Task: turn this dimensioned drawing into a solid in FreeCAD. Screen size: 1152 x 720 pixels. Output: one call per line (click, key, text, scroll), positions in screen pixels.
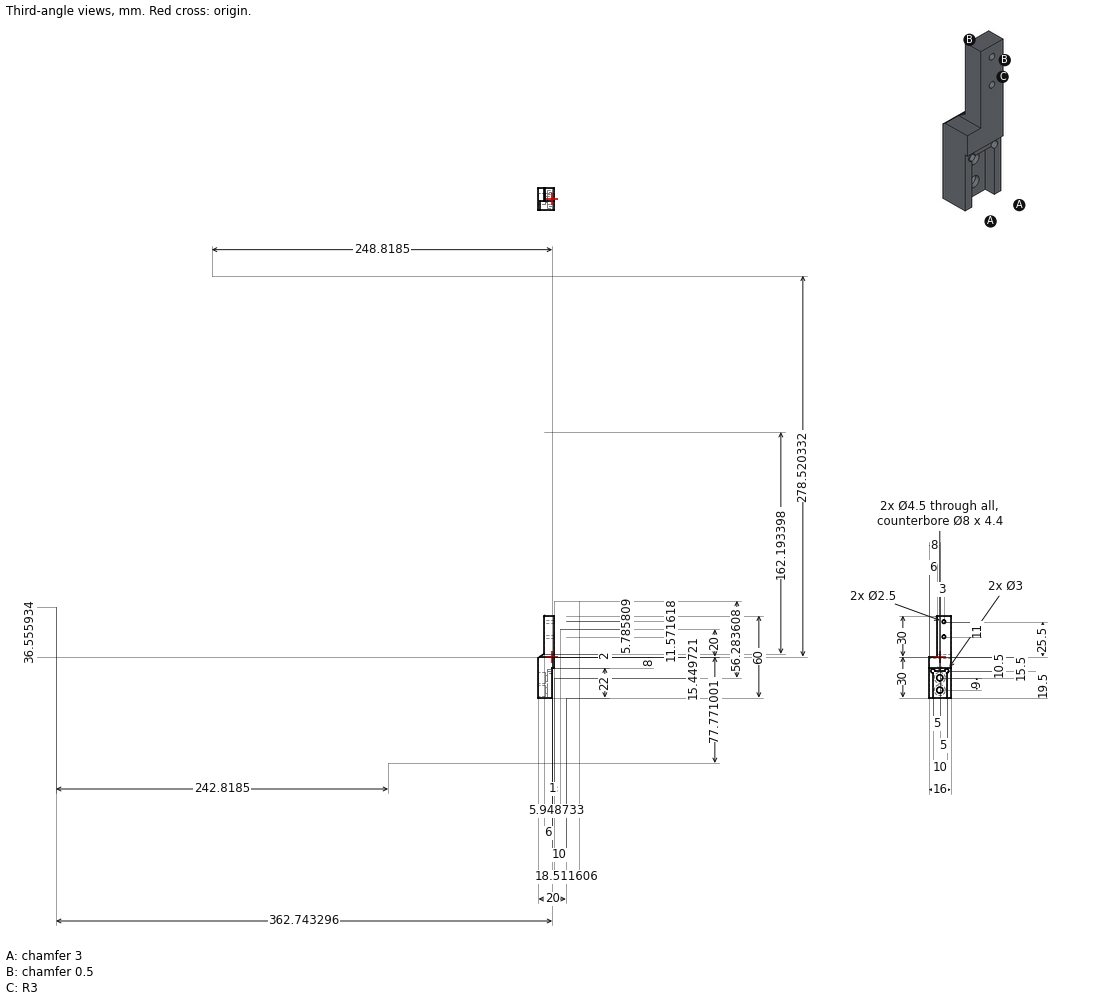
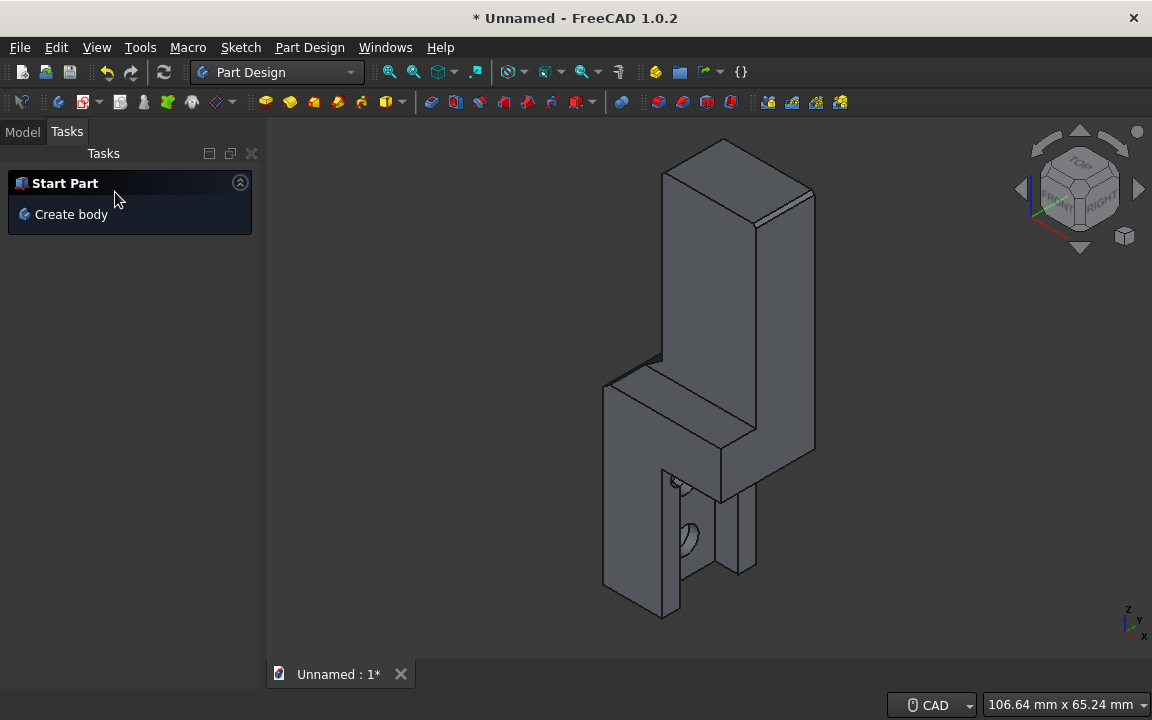
click(716, 303)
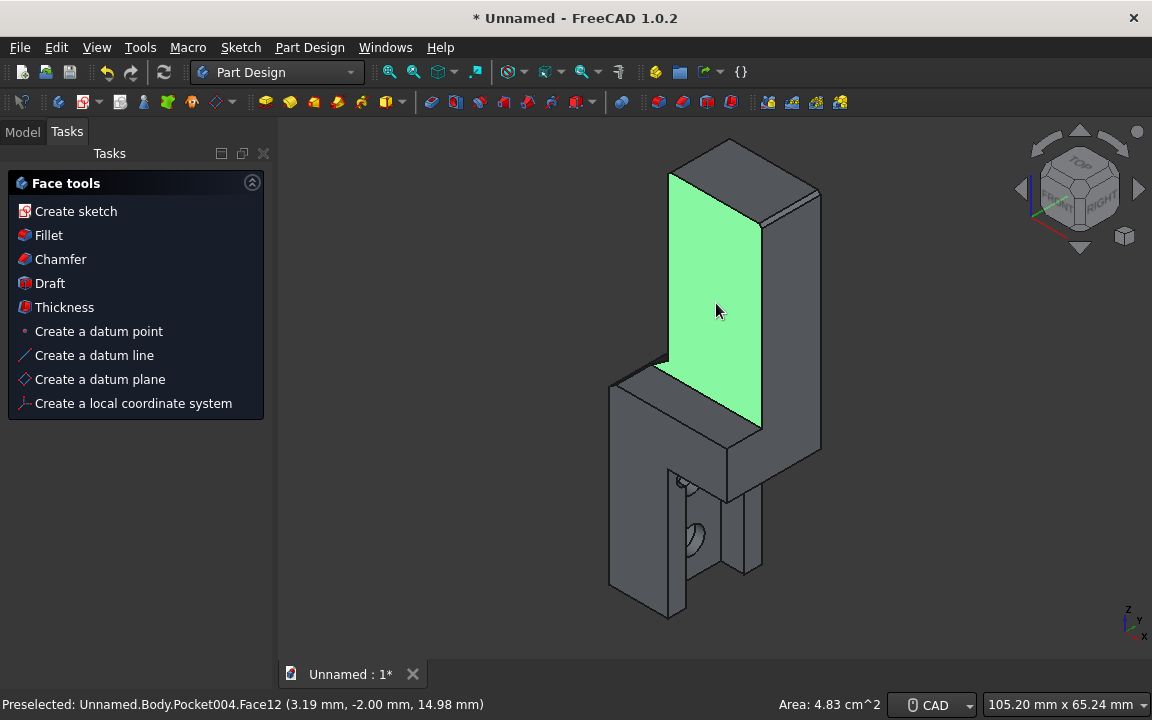
click(84, 102)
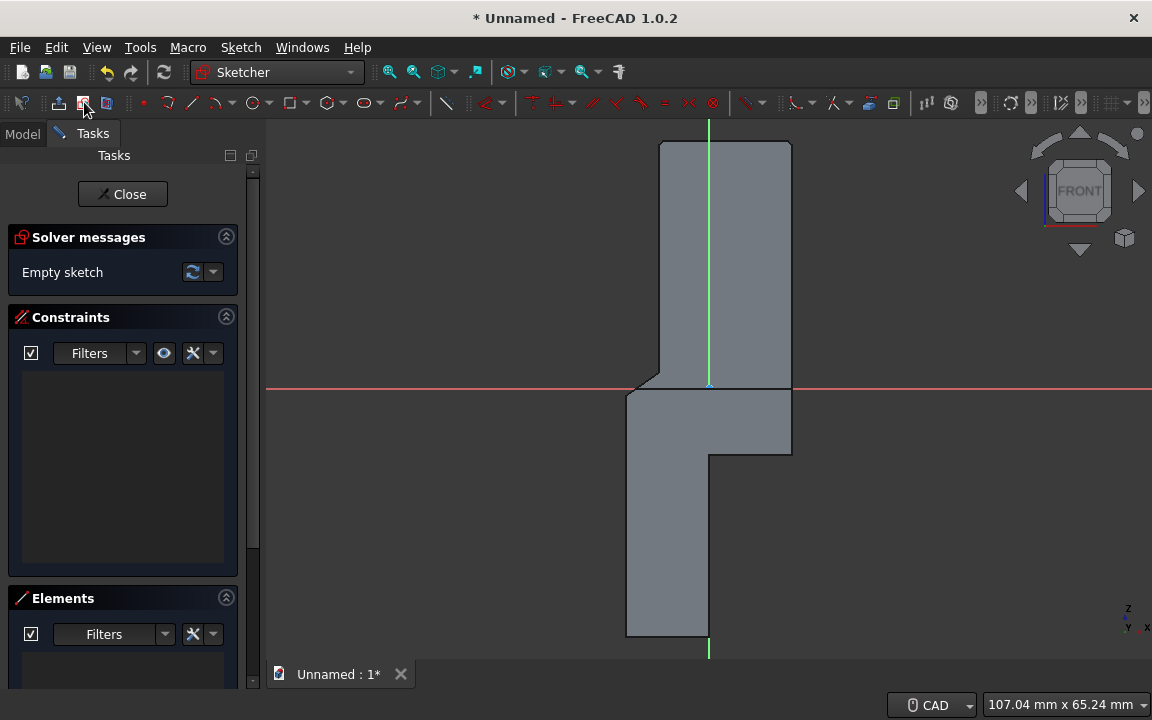
click(108, 104)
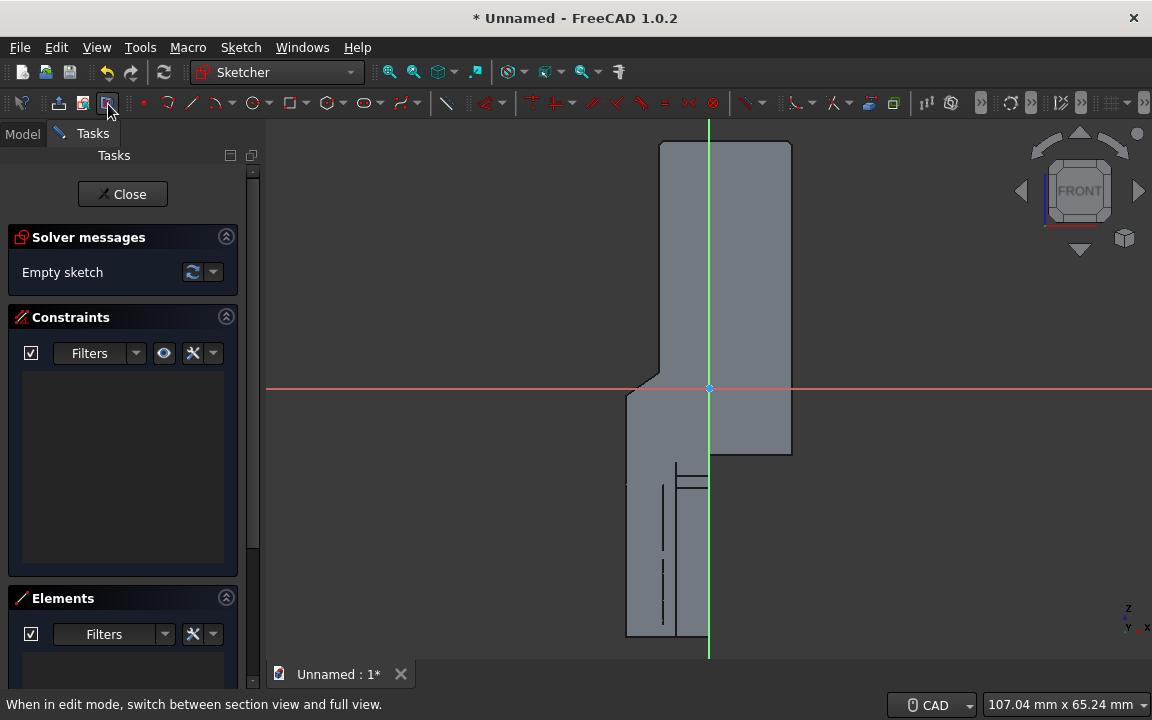
scroll(974, 147, up, 2)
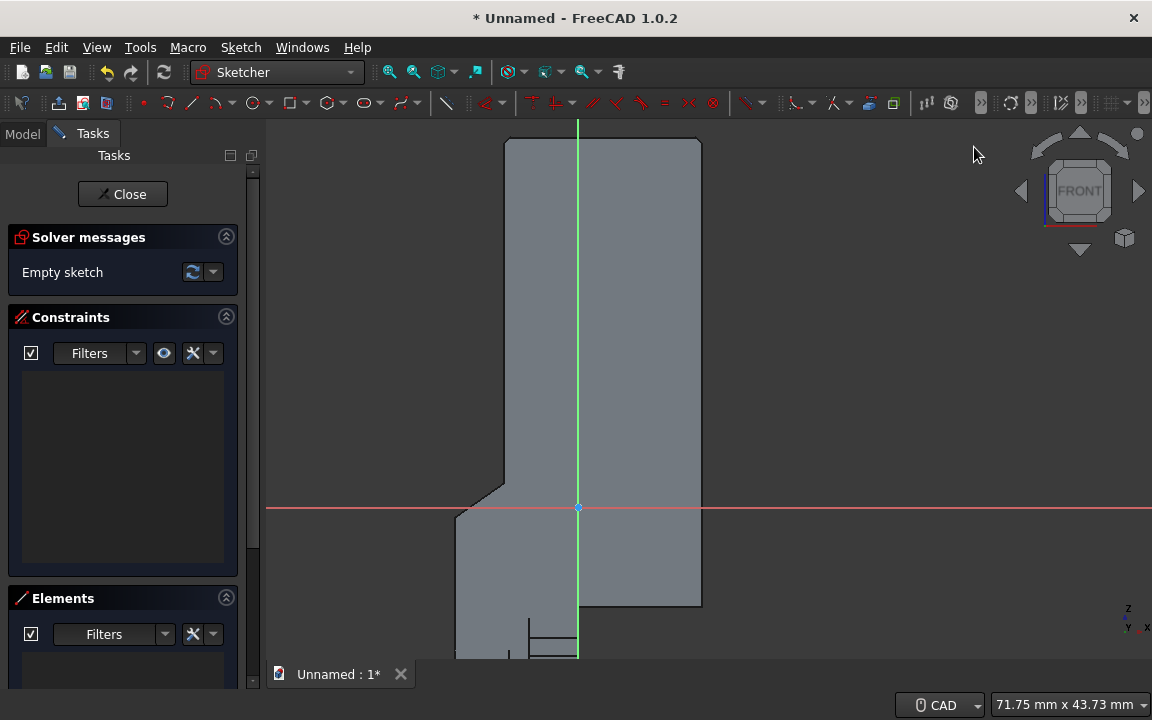
key(g)
key(m)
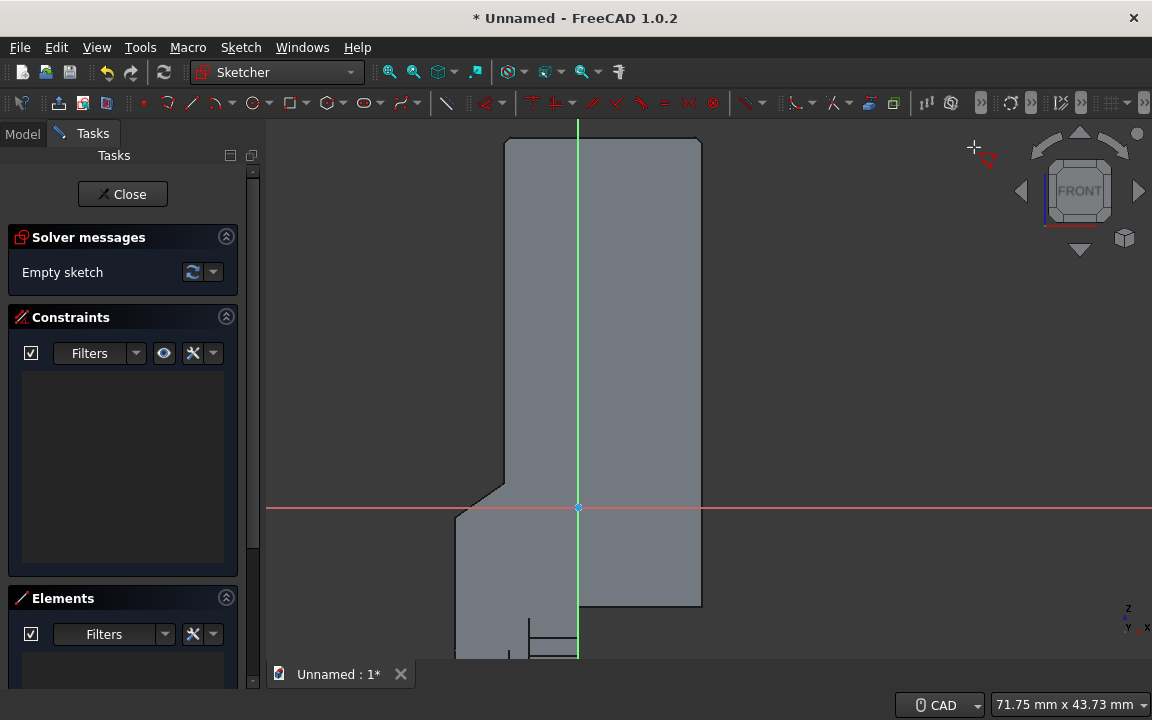
click(702, 332)
click(702, 190)
click(652, 261)
click(702, 333)
key(Escape)
key(Escape)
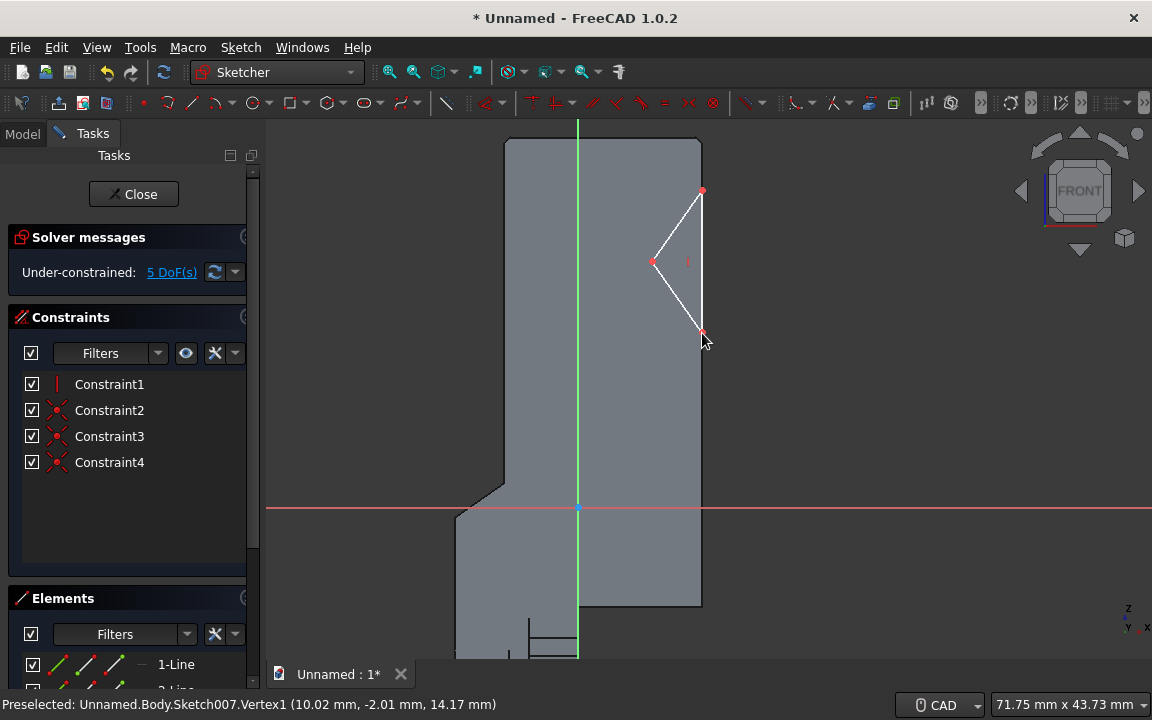
key(d)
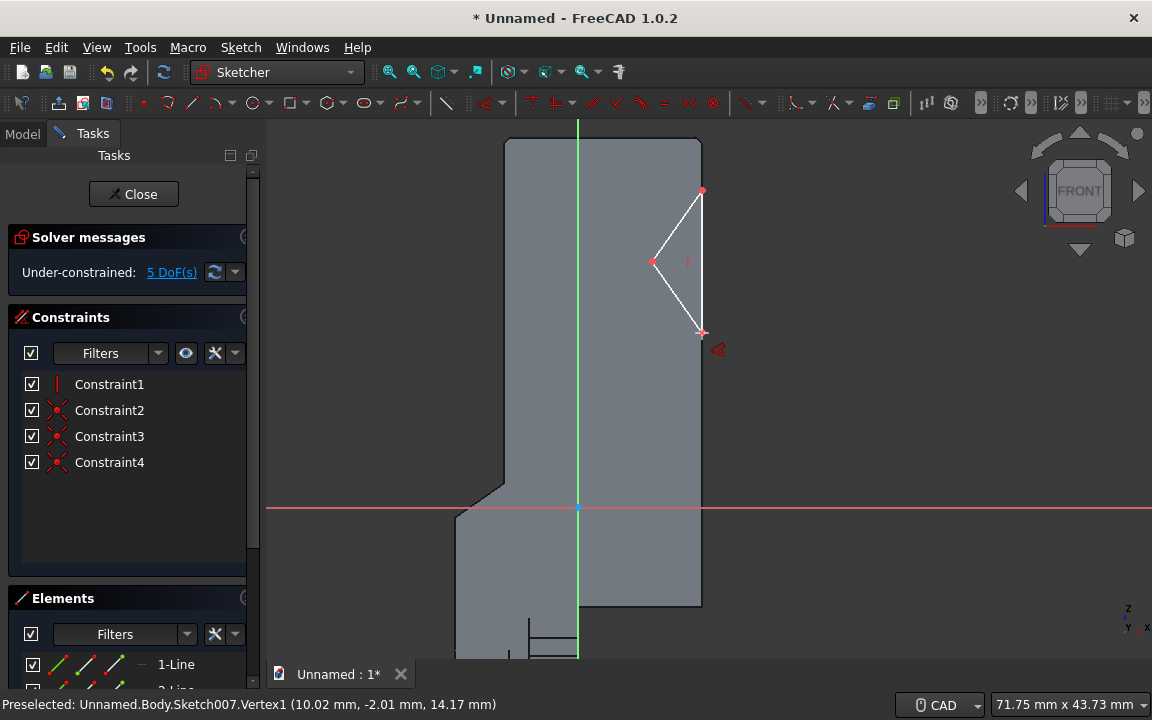
click(702, 333)
click(640, 542)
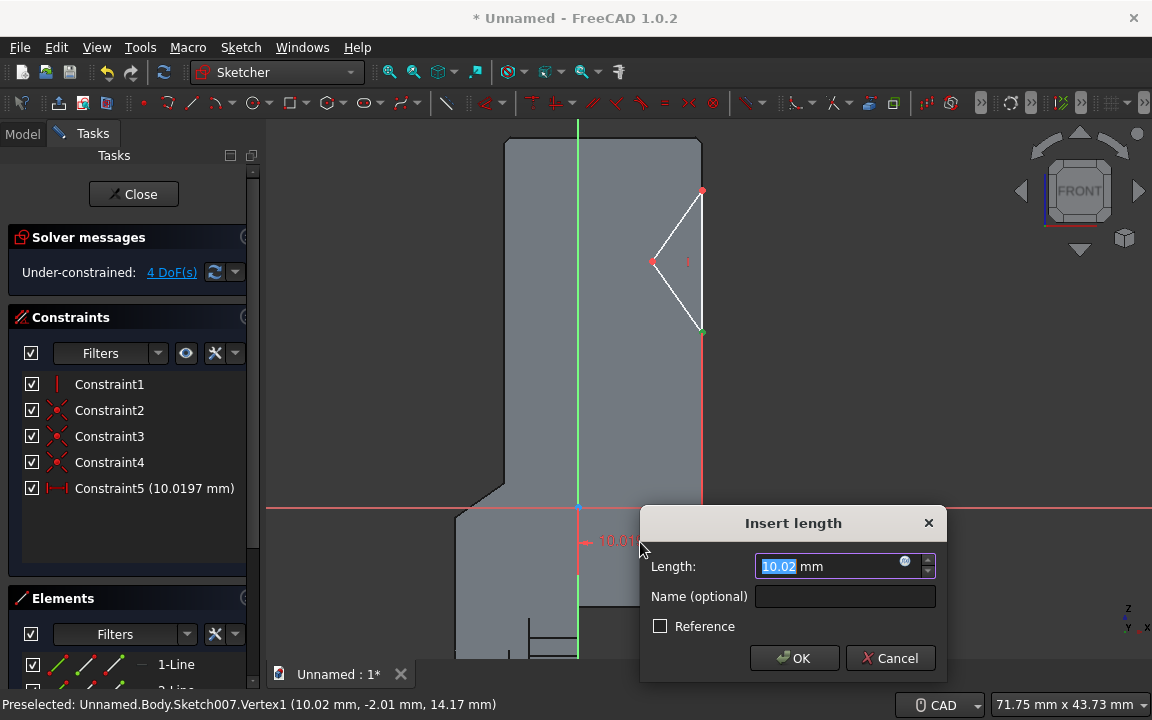
text(10)
key(Return)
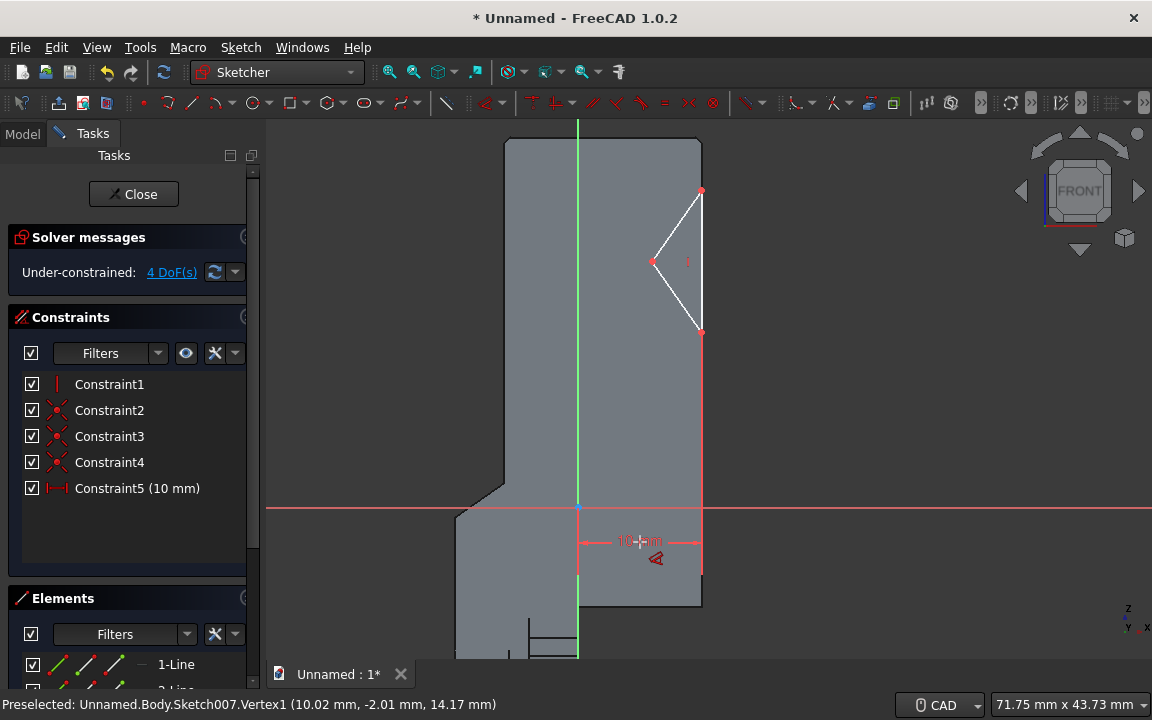
click(652, 262)
click(544, 385)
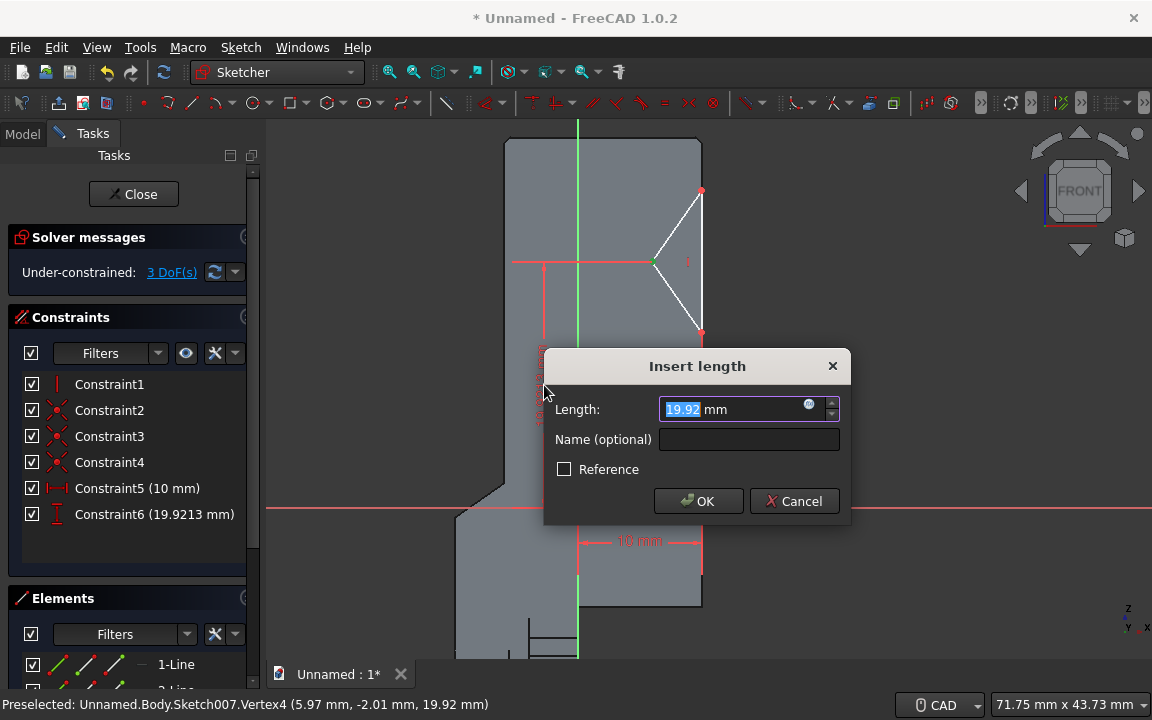
text(20)
key(Return)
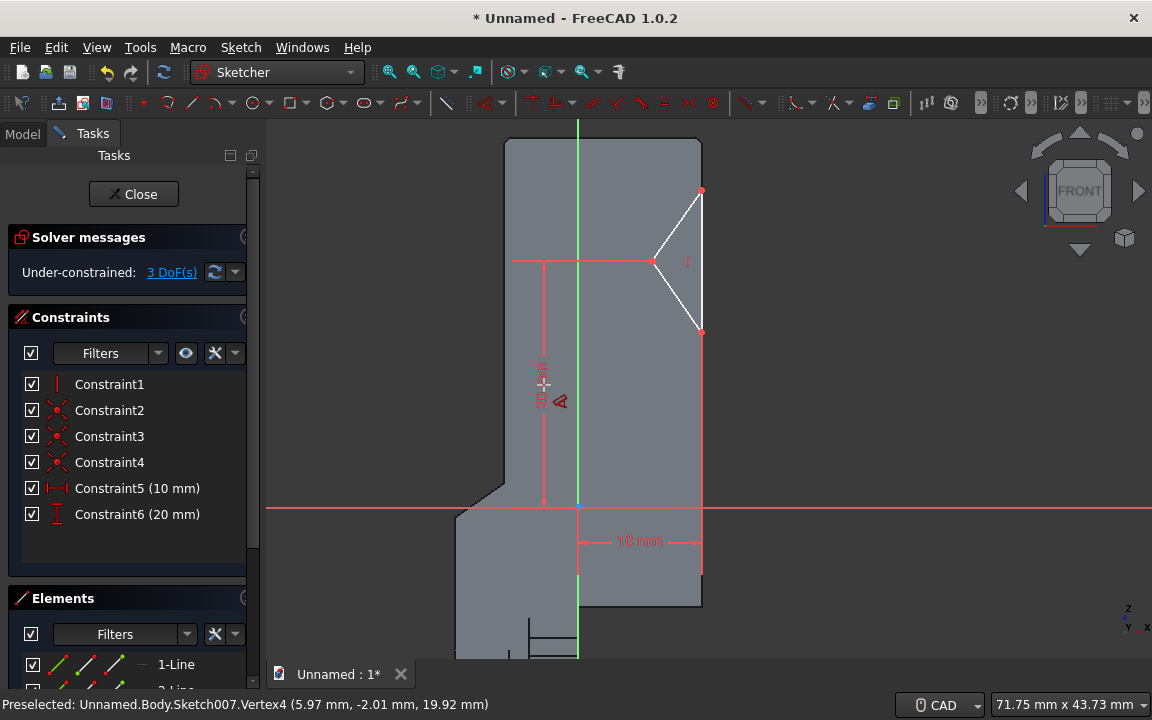
click(702, 290)
click(736, 262)